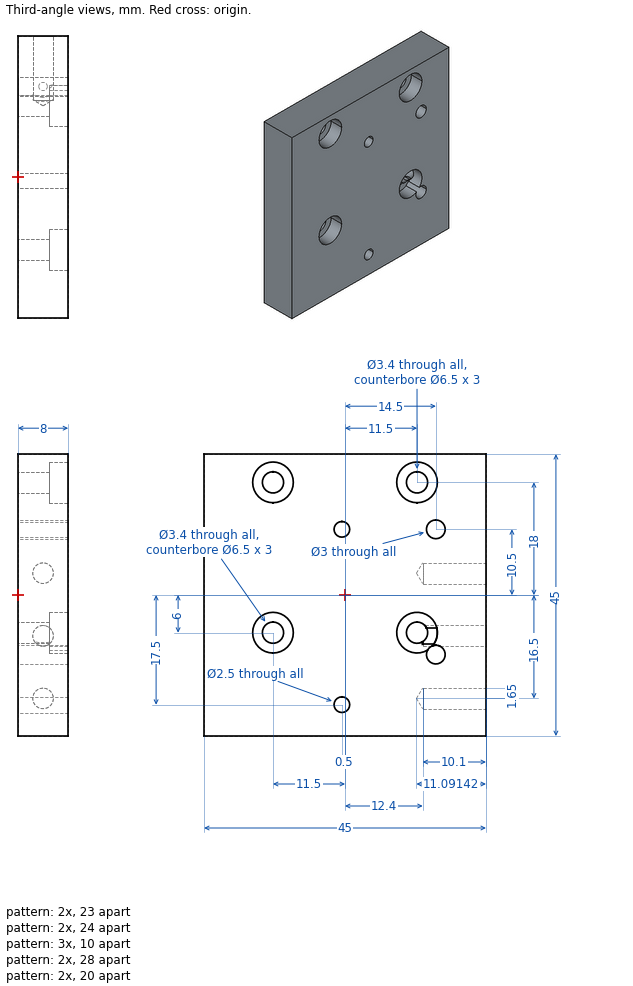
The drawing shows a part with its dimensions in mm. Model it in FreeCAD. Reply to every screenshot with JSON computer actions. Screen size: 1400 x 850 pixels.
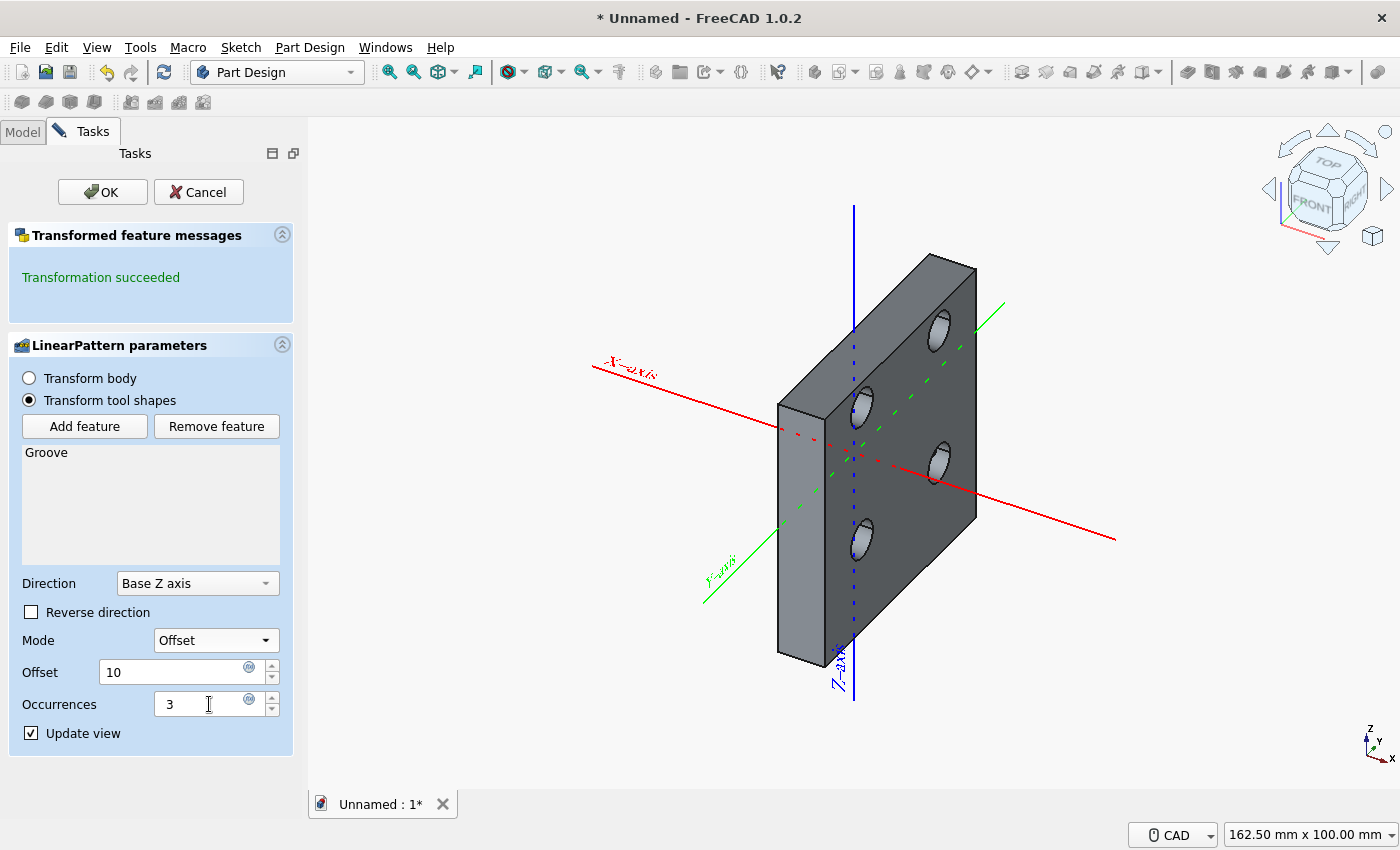
{"action": "left_click", "coordinate": [103, 192]}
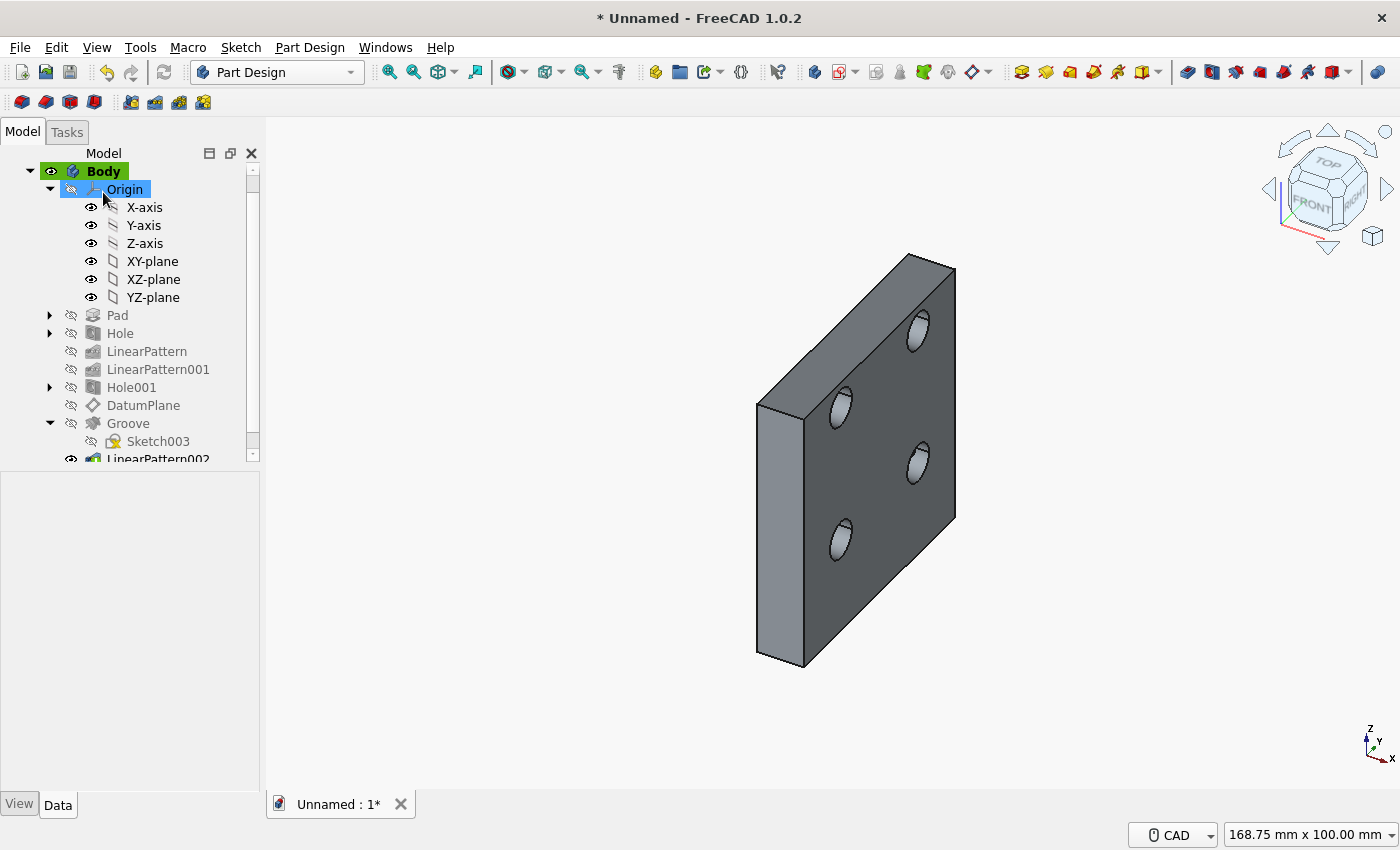
{"action": "left_click", "coordinate": [880, 432]}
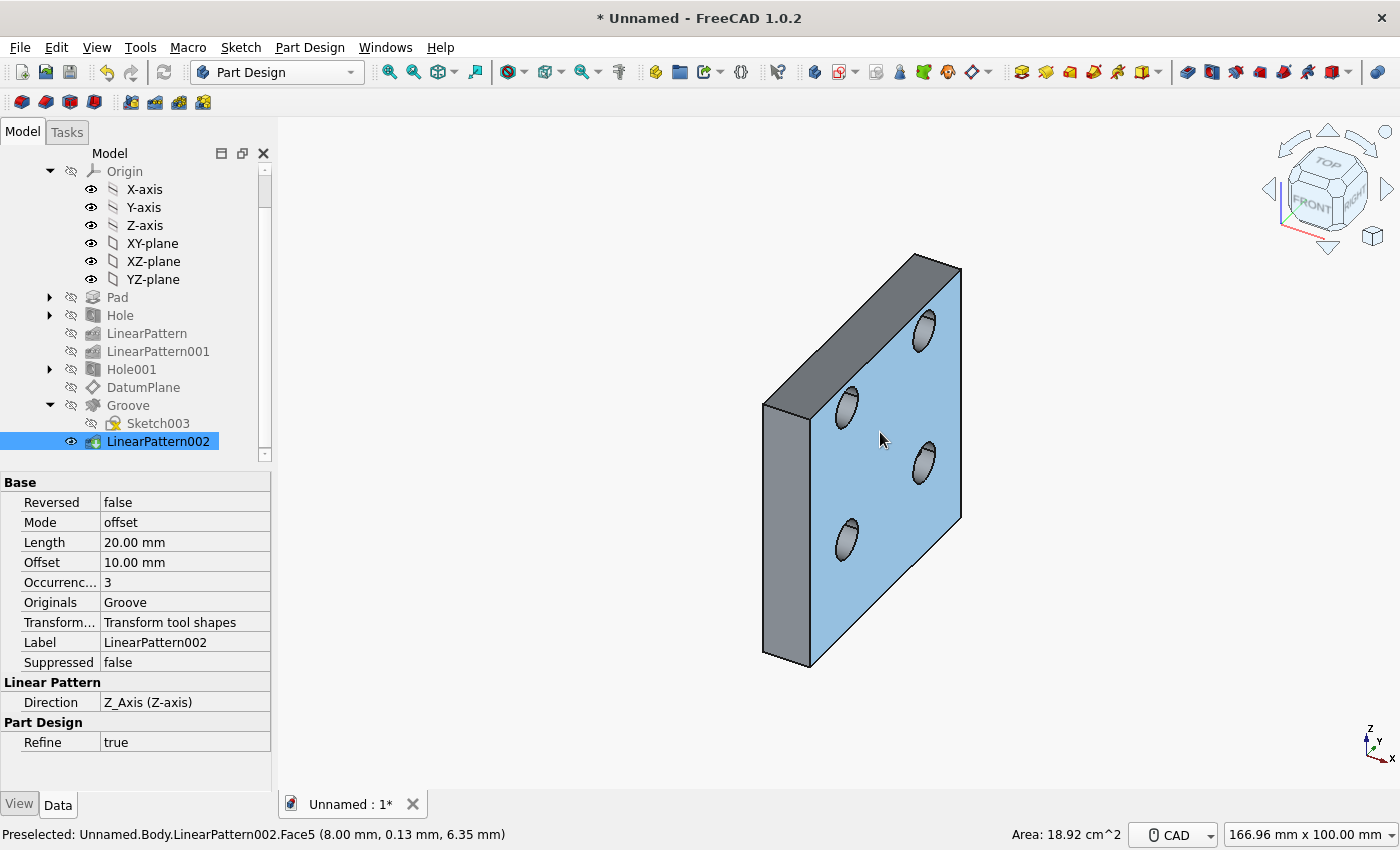
{"action": "left_click", "coordinate": [840, 72]}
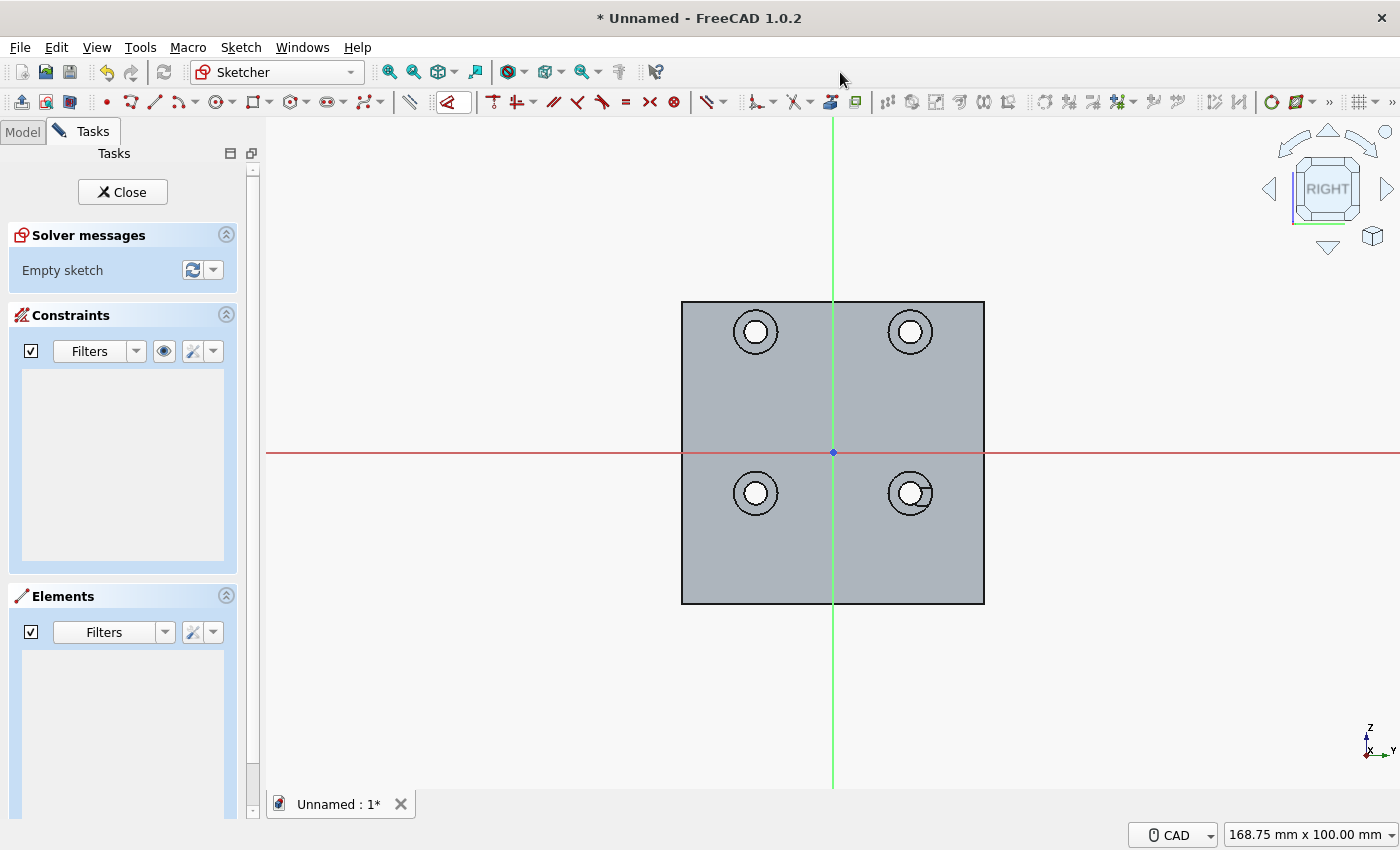
{"action": "scroll", "coordinate": [833, 577], "scroll_direction": "up", "scroll_amount": 15}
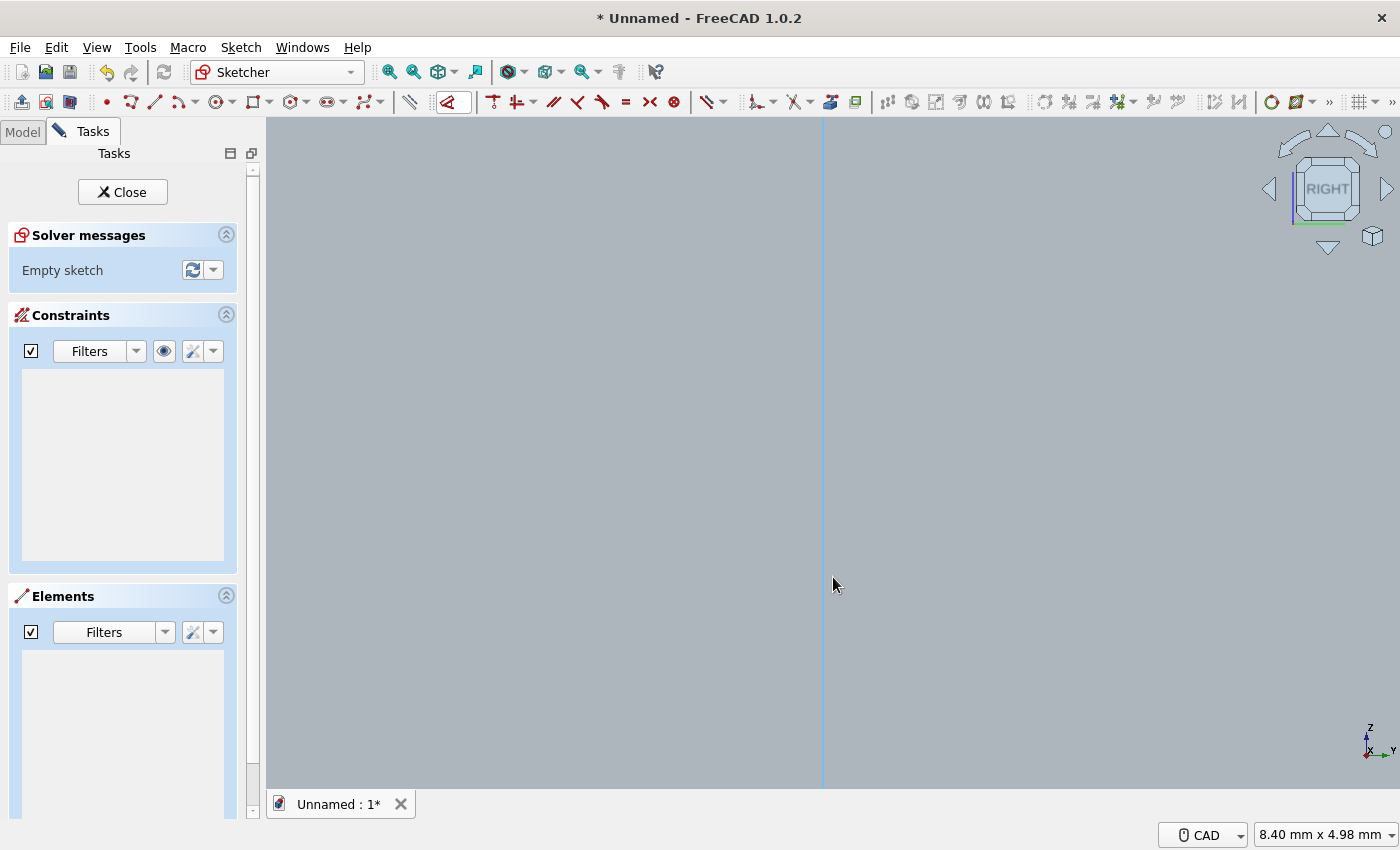
{"action": "key", "text": "g c"}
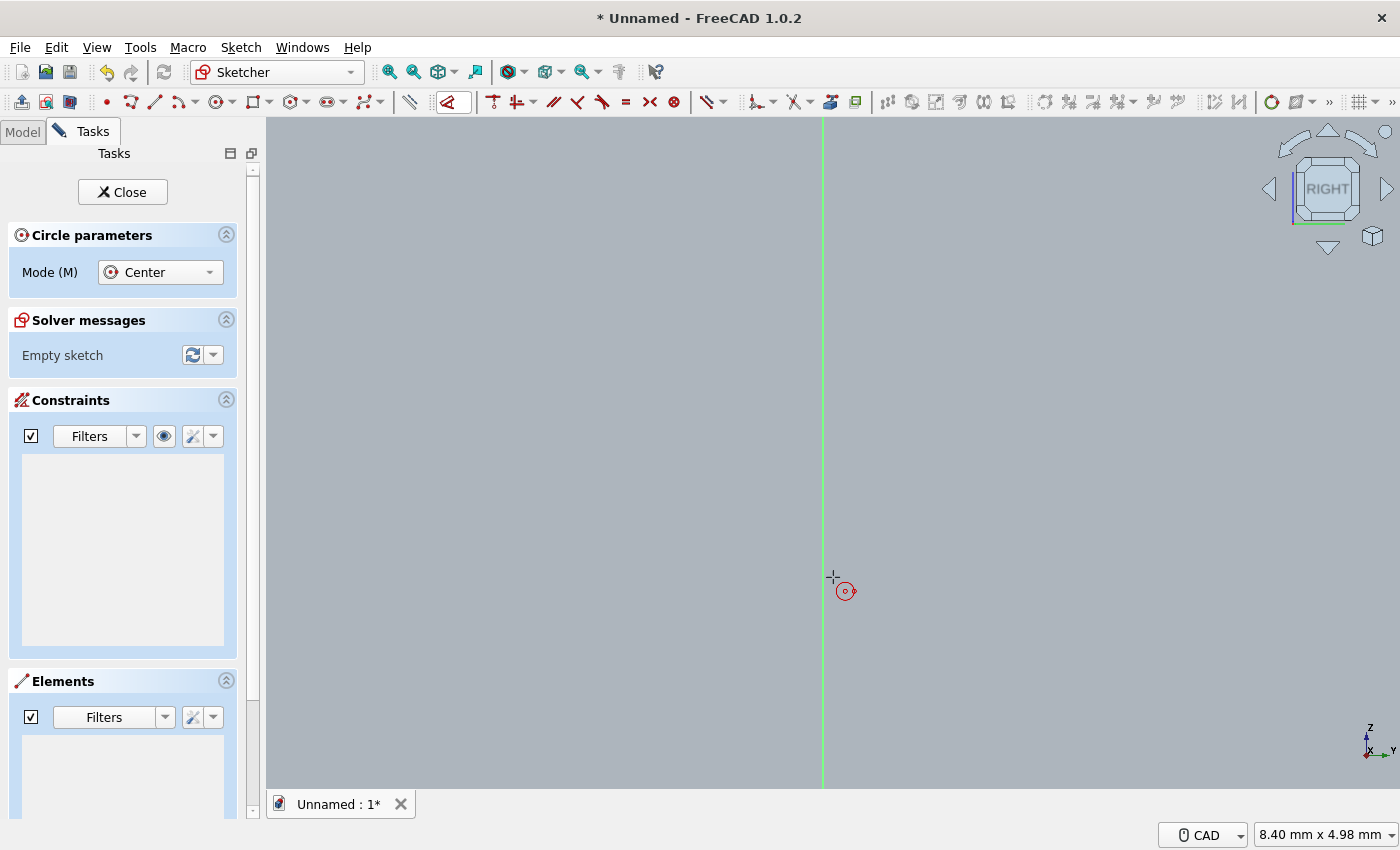
{"action": "left_click", "coordinate": [756, 435]}
{"action": "left_click", "coordinate": [875, 316]}
{"action": "key", "text": "Escape"}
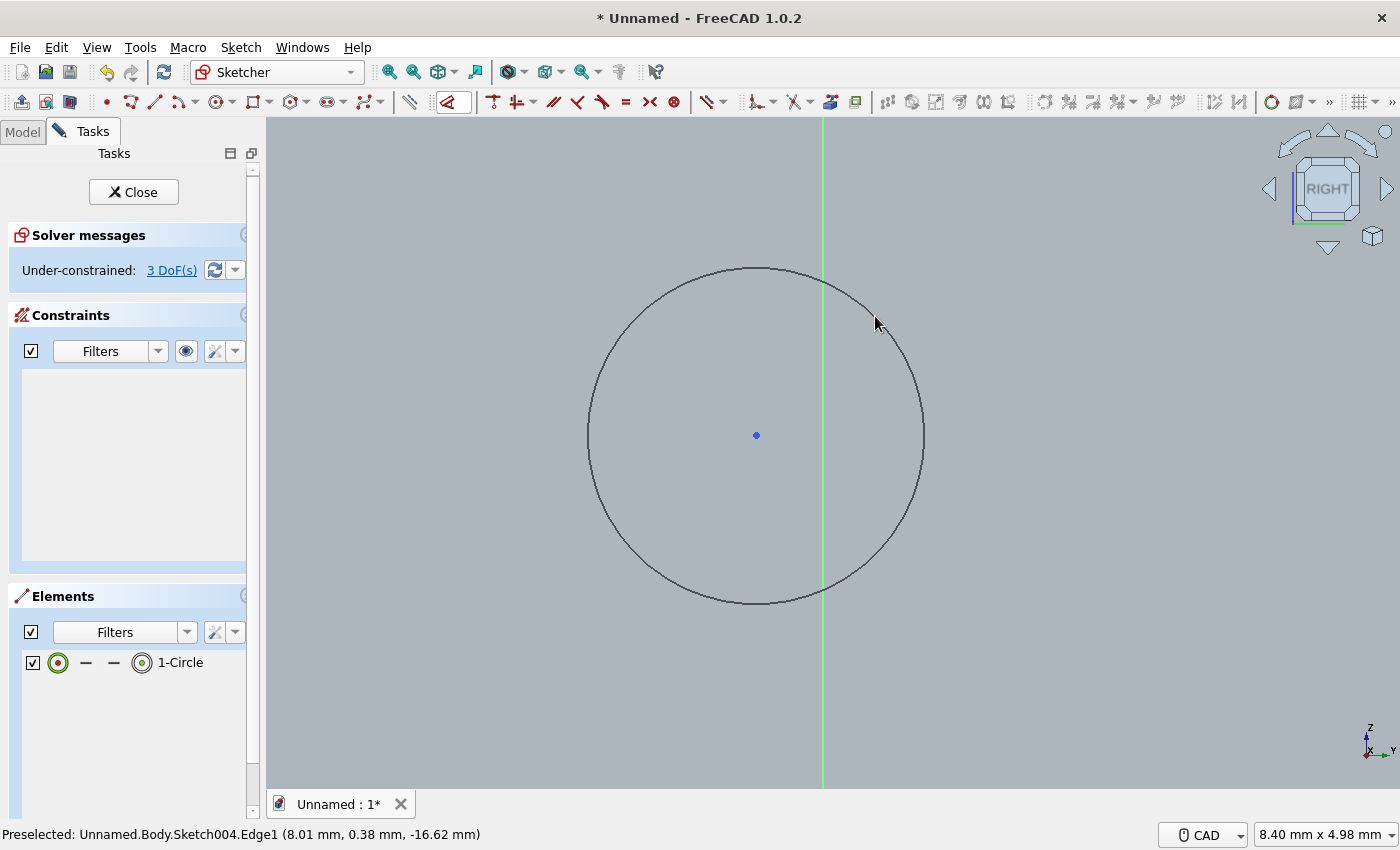
{"action": "left_click", "coordinate": [448, 102]}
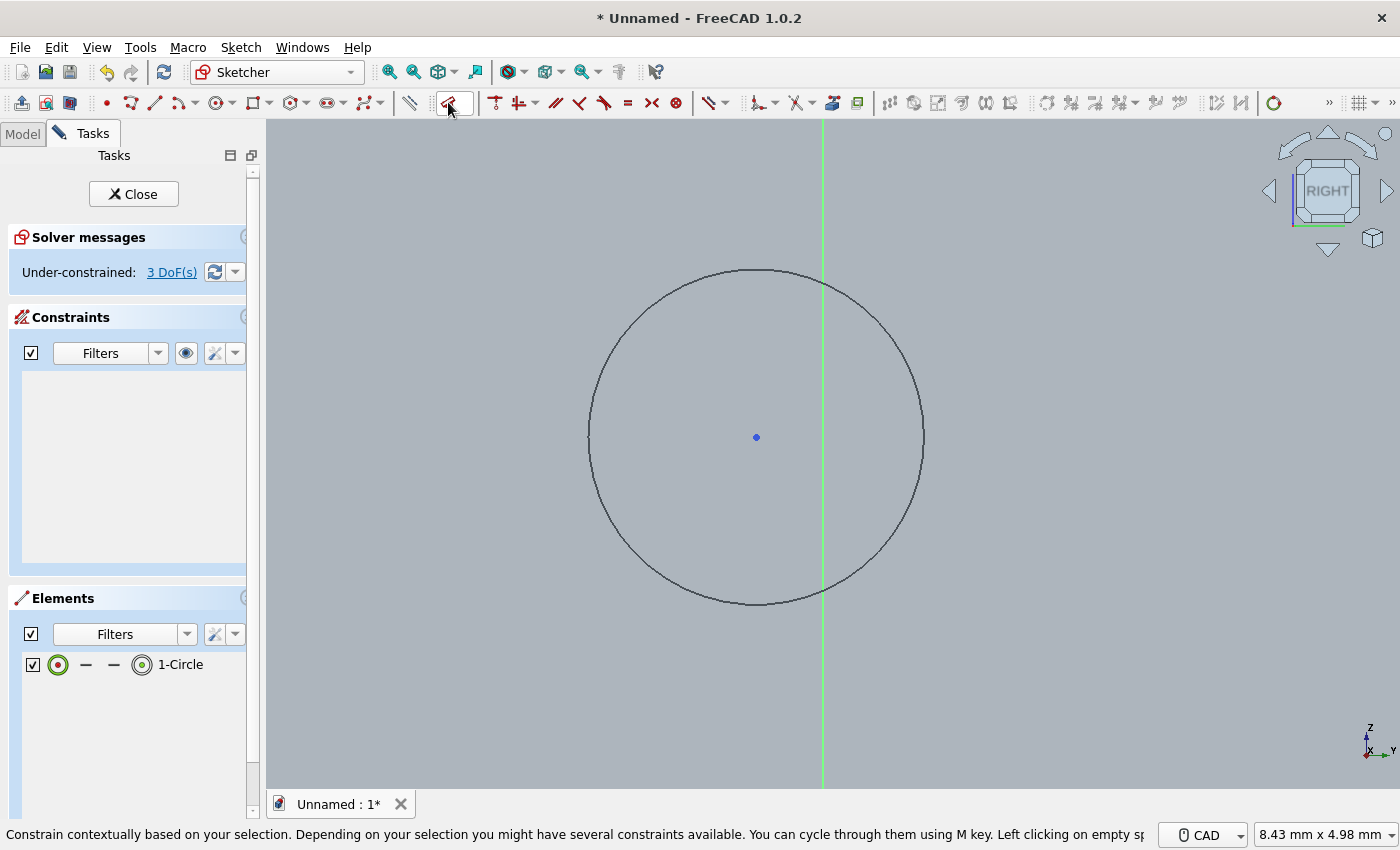
{"action": "left_click", "coordinate": [875, 318]}
{"action": "left_click", "coordinate": [898, 295]}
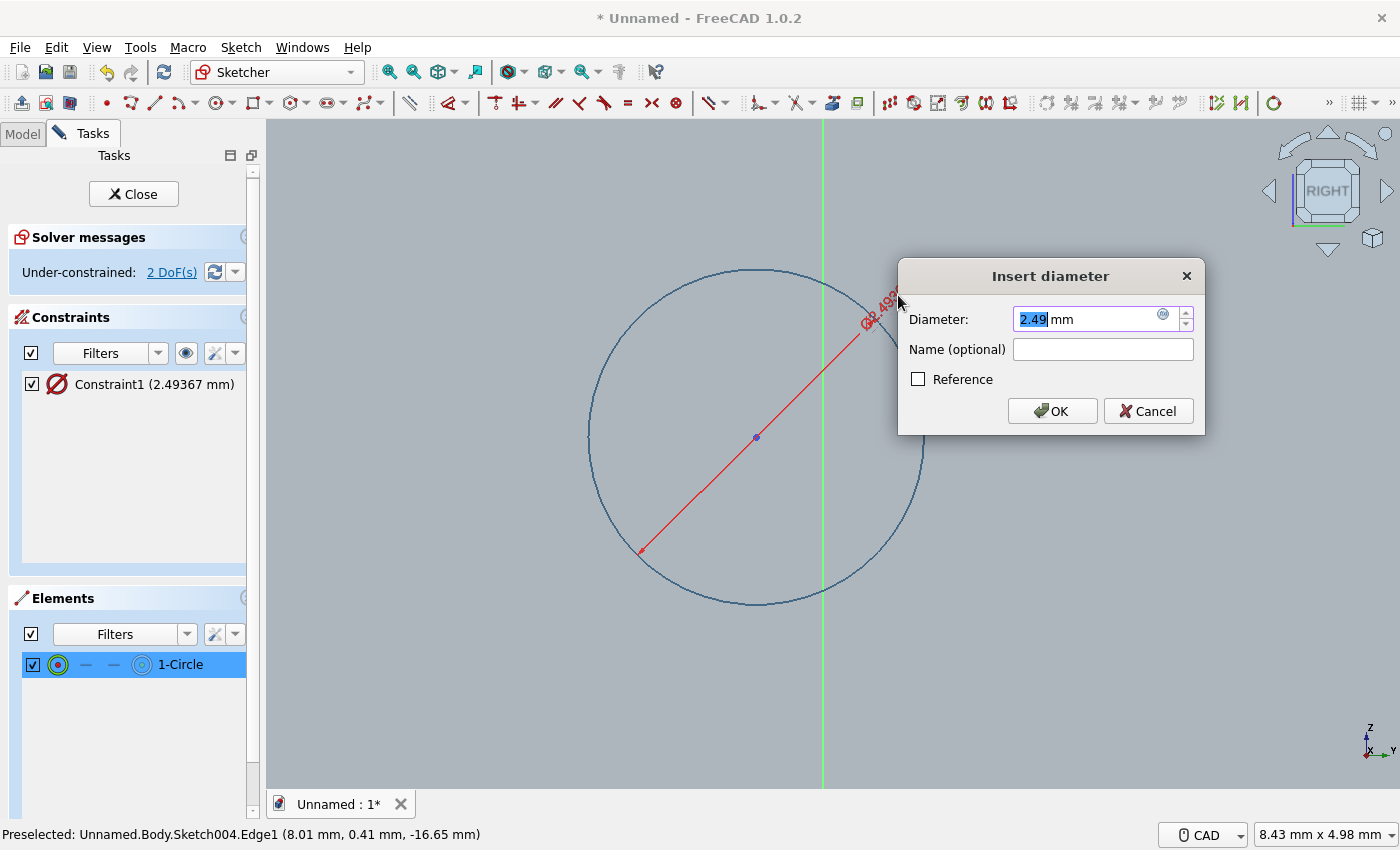
{"action": "type", "text": "2.5"}
{"action": "key", "text": "Return"}